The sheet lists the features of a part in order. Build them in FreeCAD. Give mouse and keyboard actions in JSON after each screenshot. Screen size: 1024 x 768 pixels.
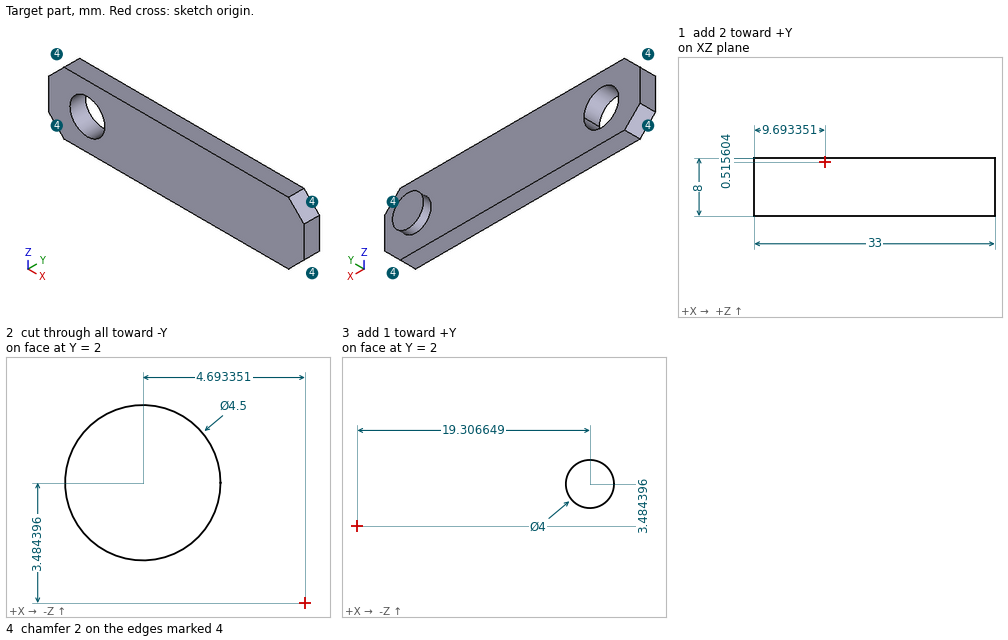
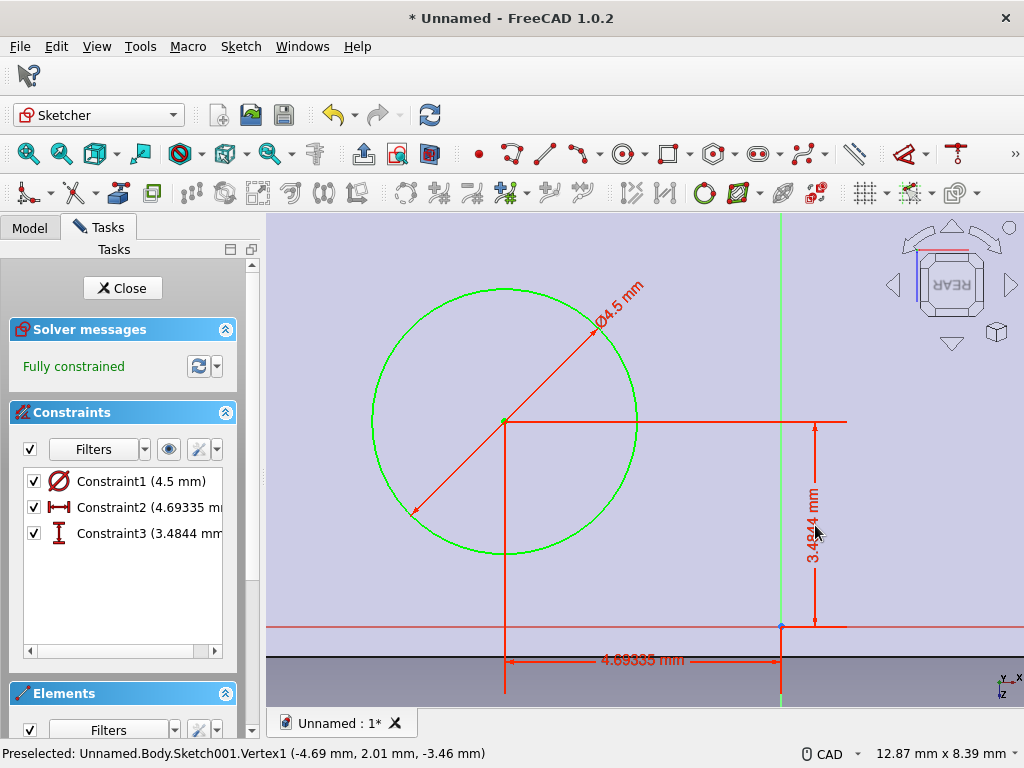
{"action": "left_click", "coordinate": [123, 288]}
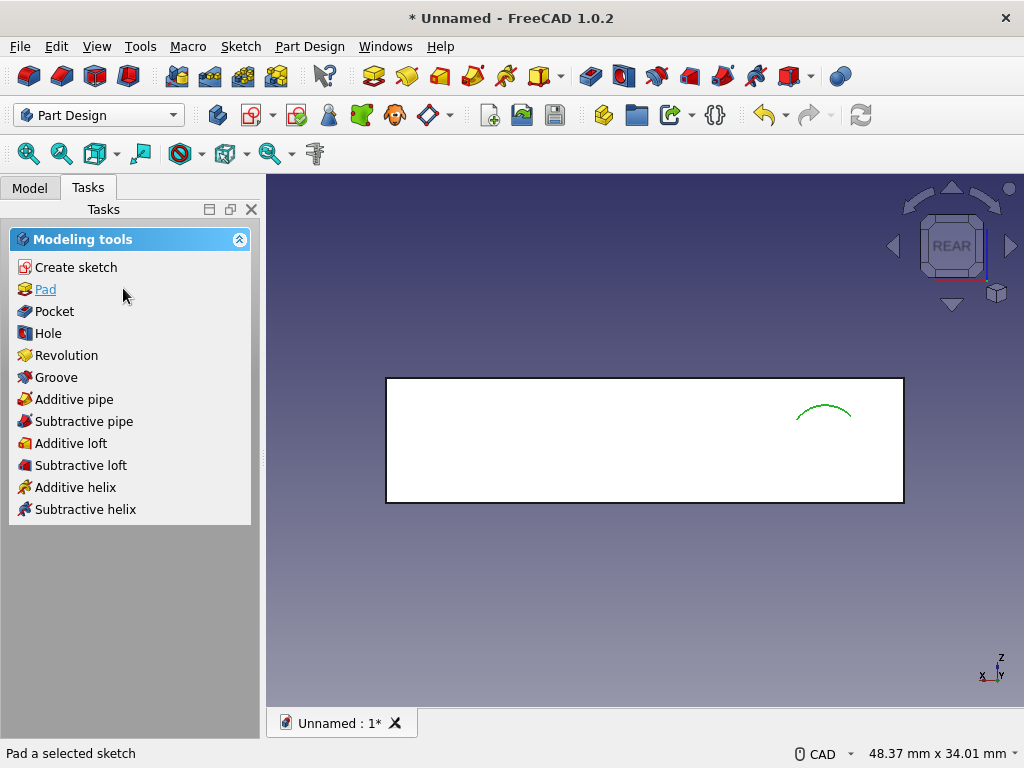
{"action": "left_click", "coordinate": [591, 76]}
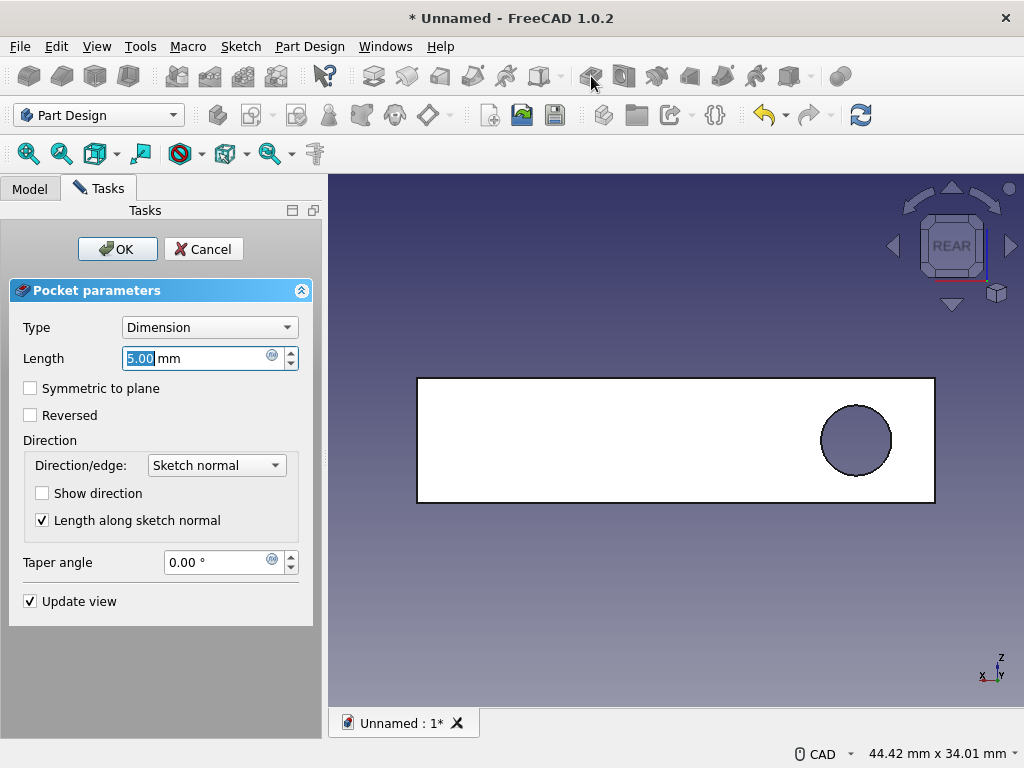
{"action": "left_click", "coordinate": [210, 328]}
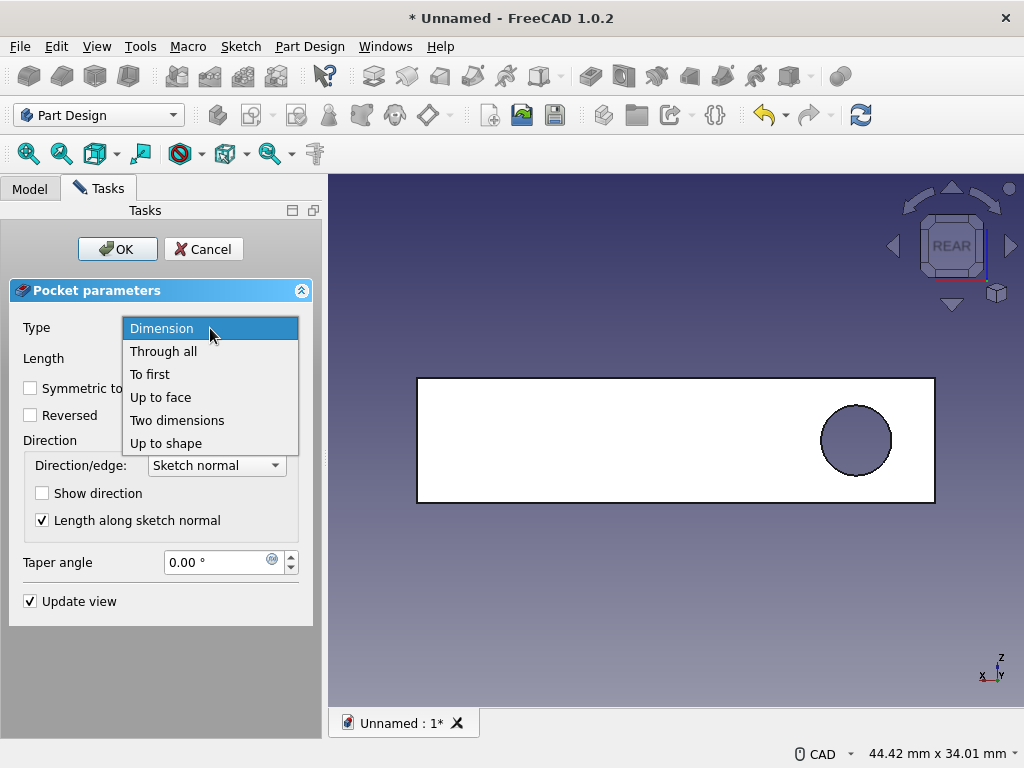
{"action": "left_click", "coordinate": [208, 352]}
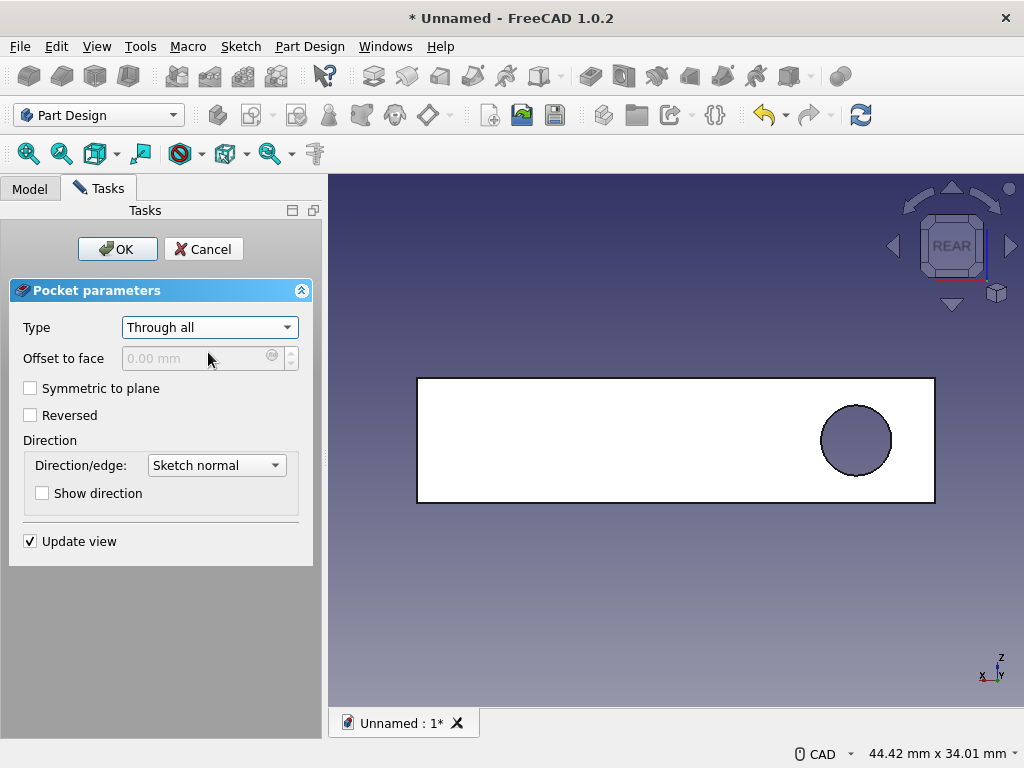
{"action": "left_click", "coordinate": [118, 249]}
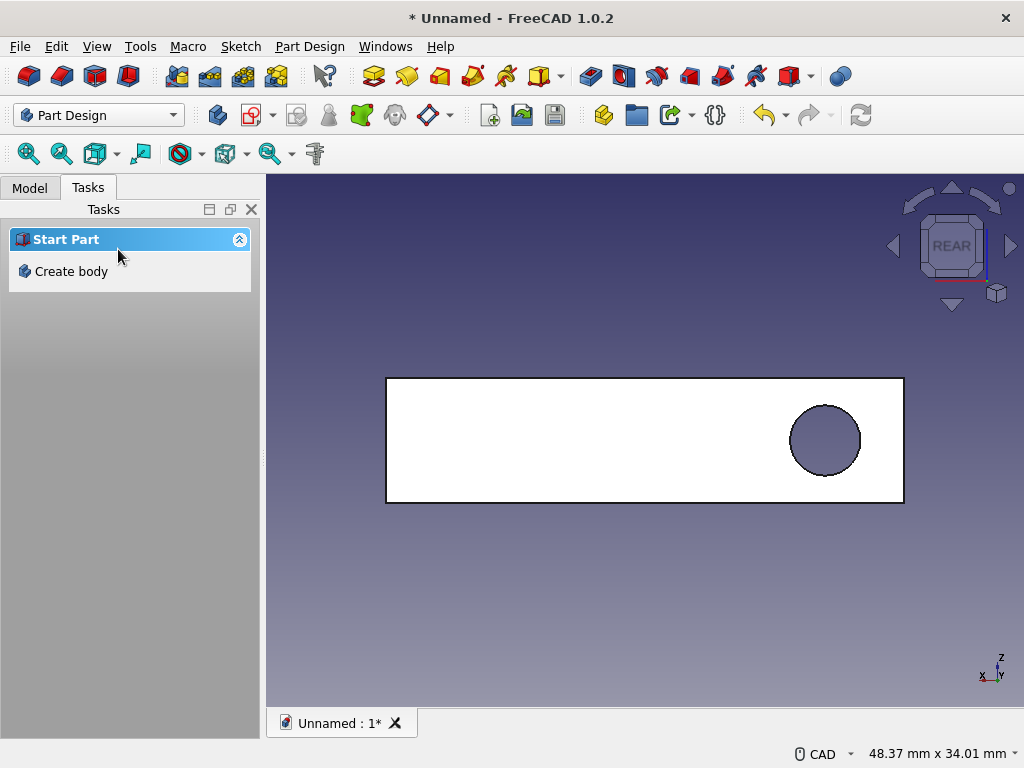
{"action": "left_click", "coordinate": [497, 439]}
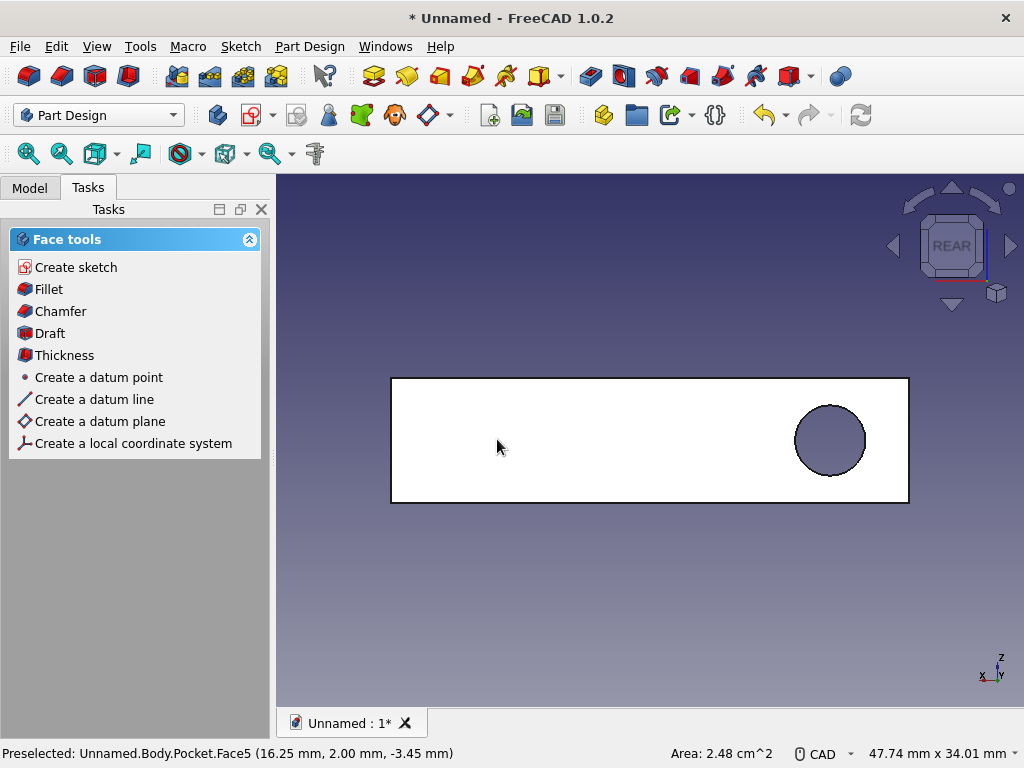
{"action": "left_click", "coordinate": [250, 116]}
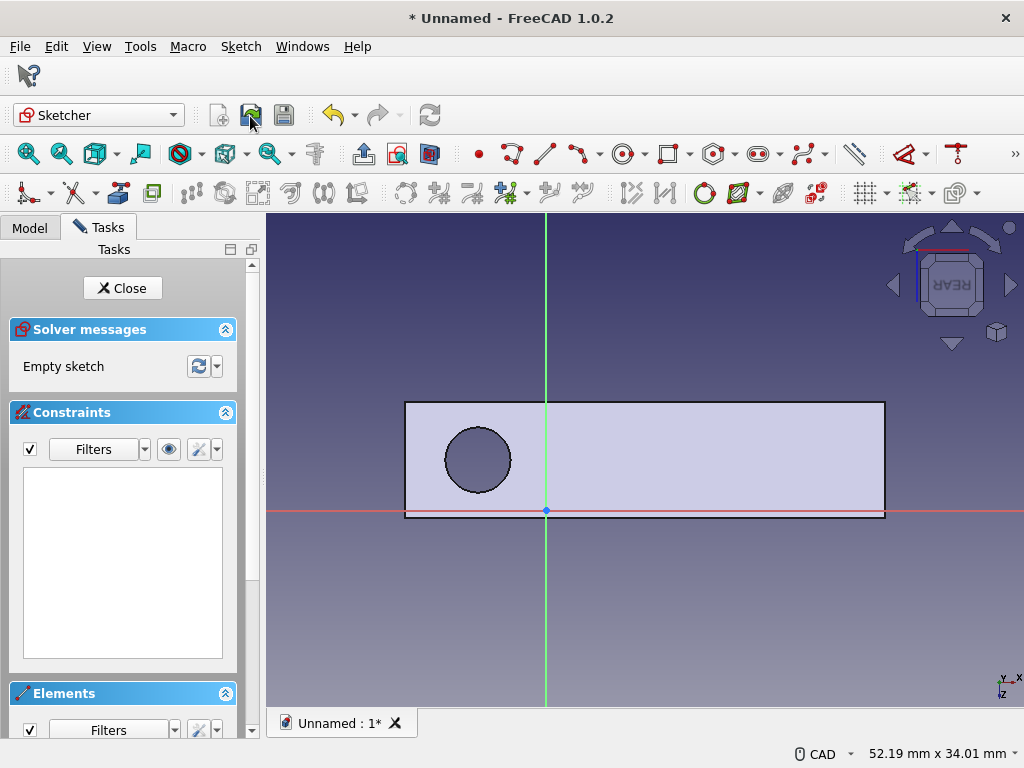
{"action": "scroll", "coordinate": [576, 460], "scroll_direction": "down", "scroll_amount": 5}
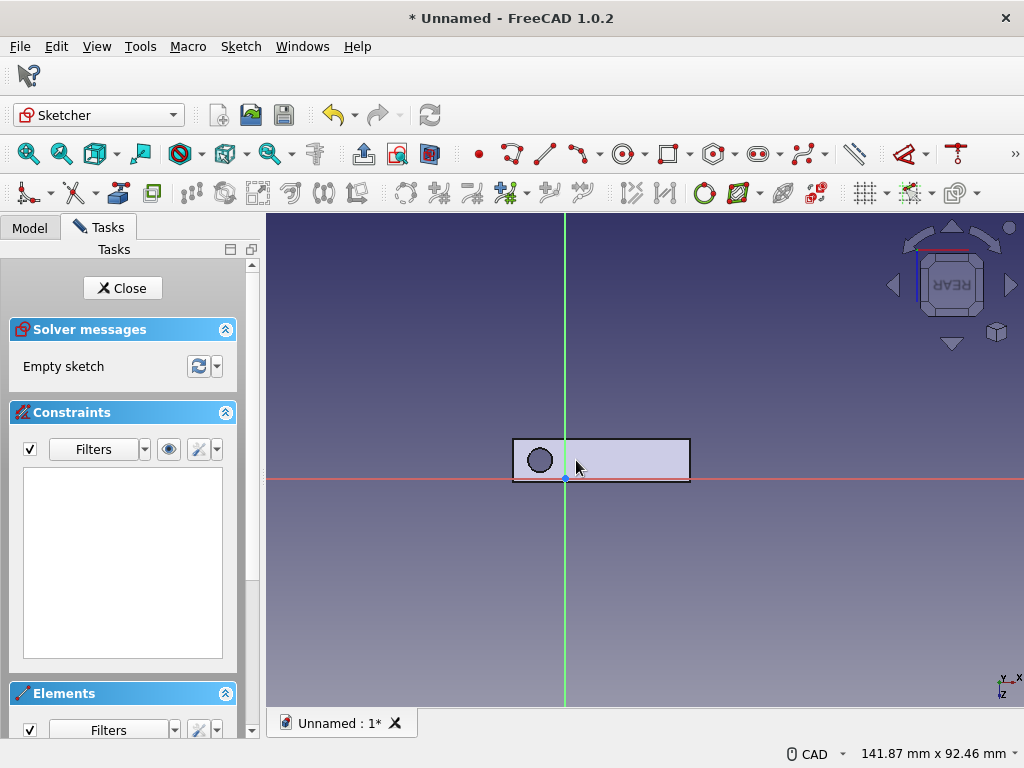
{"action": "scroll", "coordinate": [676, 460], "scroll_direction": "up", "scroll_amount": 13}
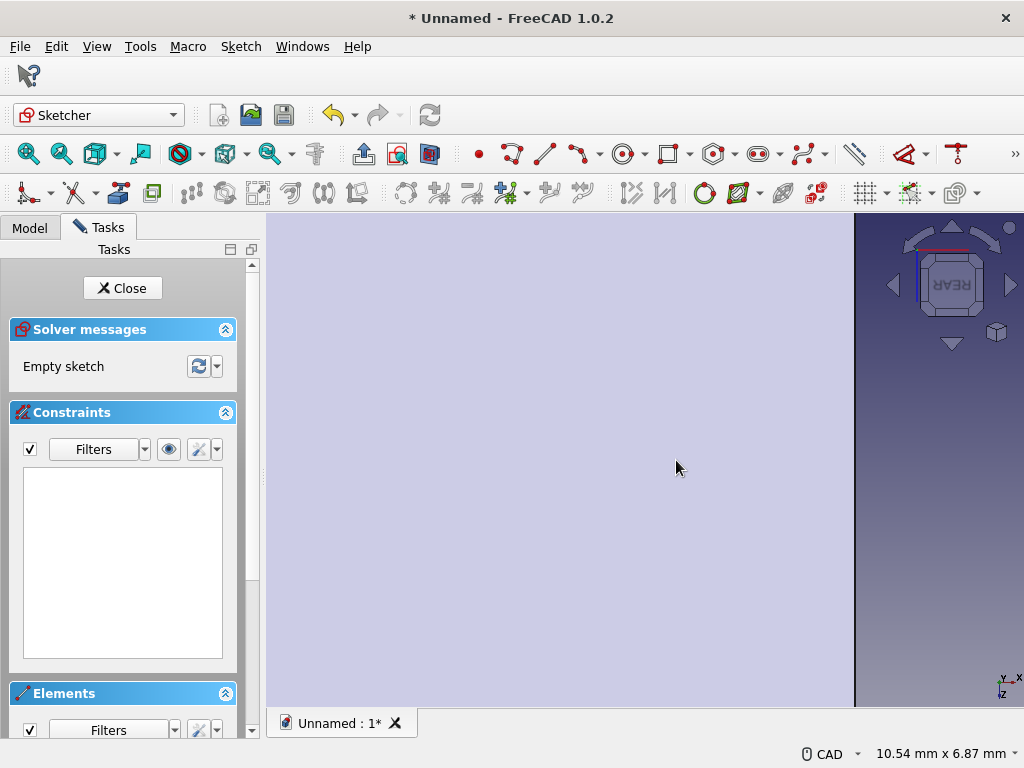
{"action": "left_click", "coordinate": [622, 154]}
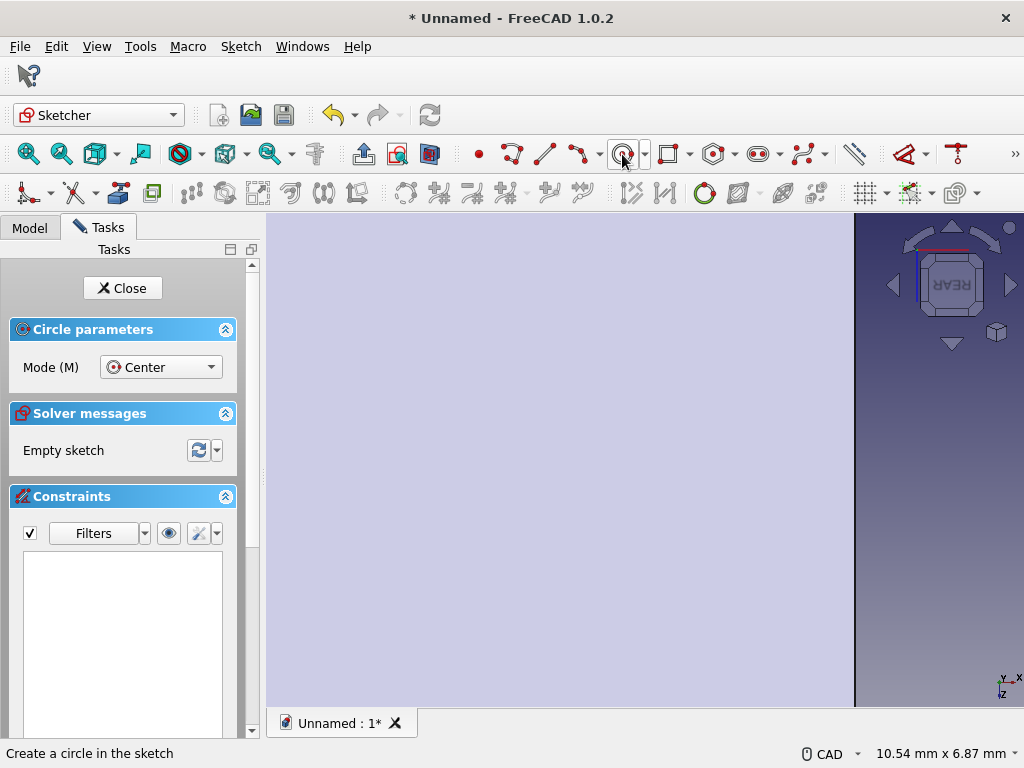
{"action": "left_click", "coordinate": [567, 458]}
{"action": "left_click", "coordinate": [669, 356]}
{"action": "key", "text": "Escape"}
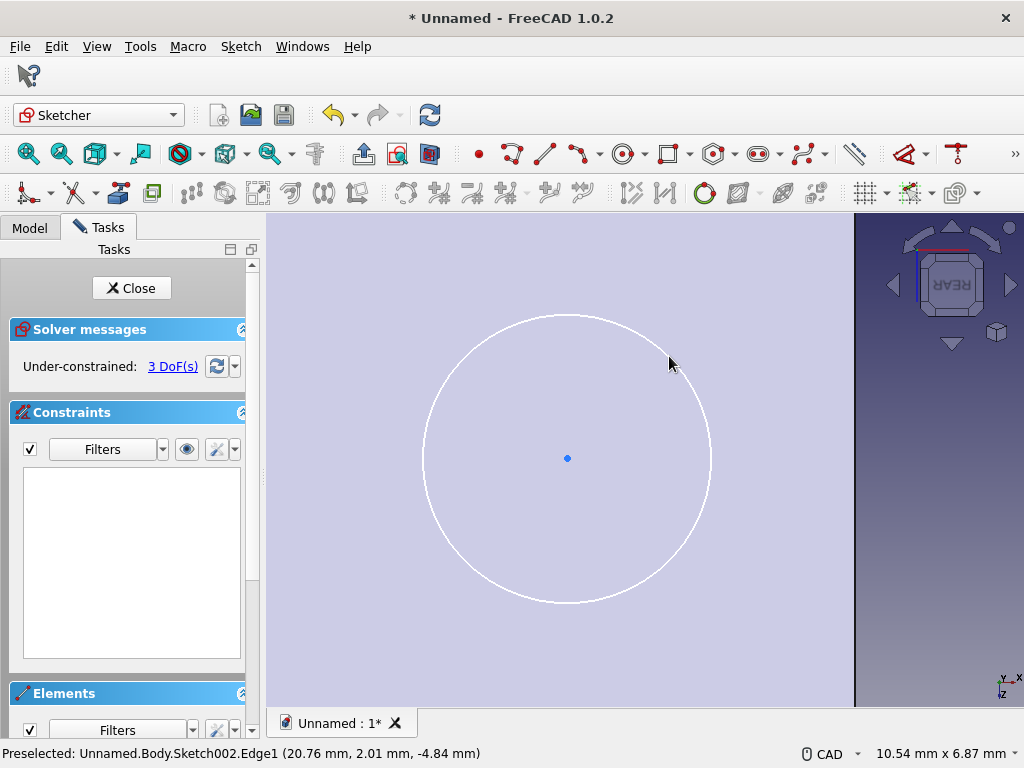
{"action": "left_click", "coordinate": [904, 154]}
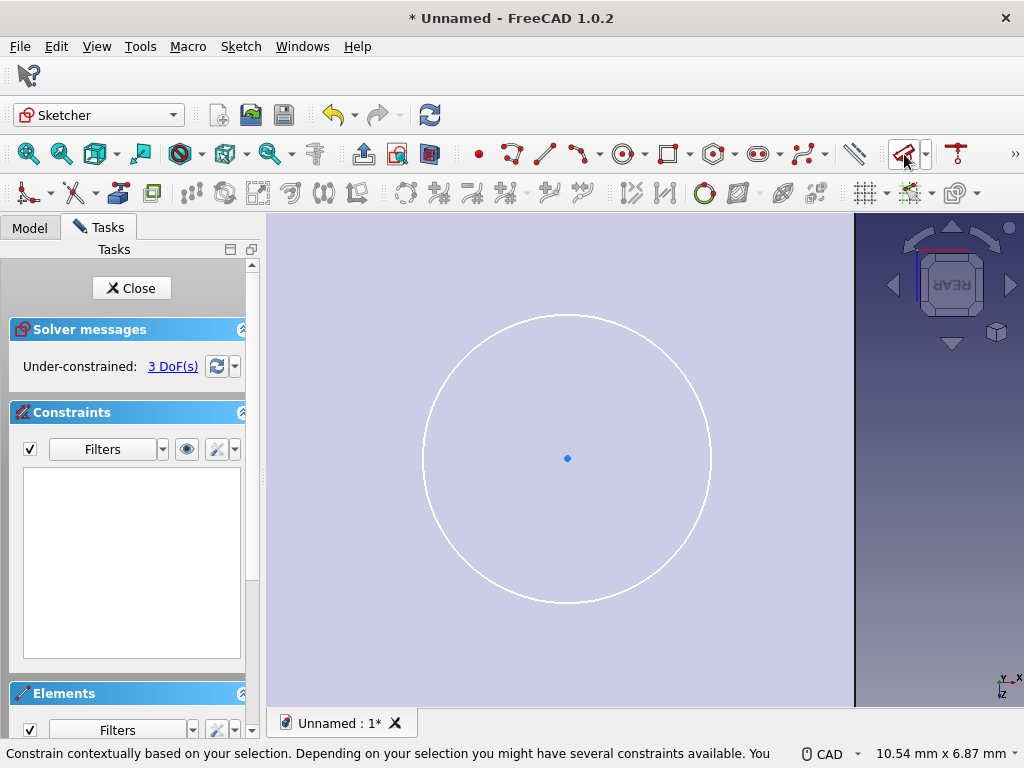
{"action": "left_click", "coordinate": [669, 357]}
{"action": "left_click", "coordinate": [692, 334]}